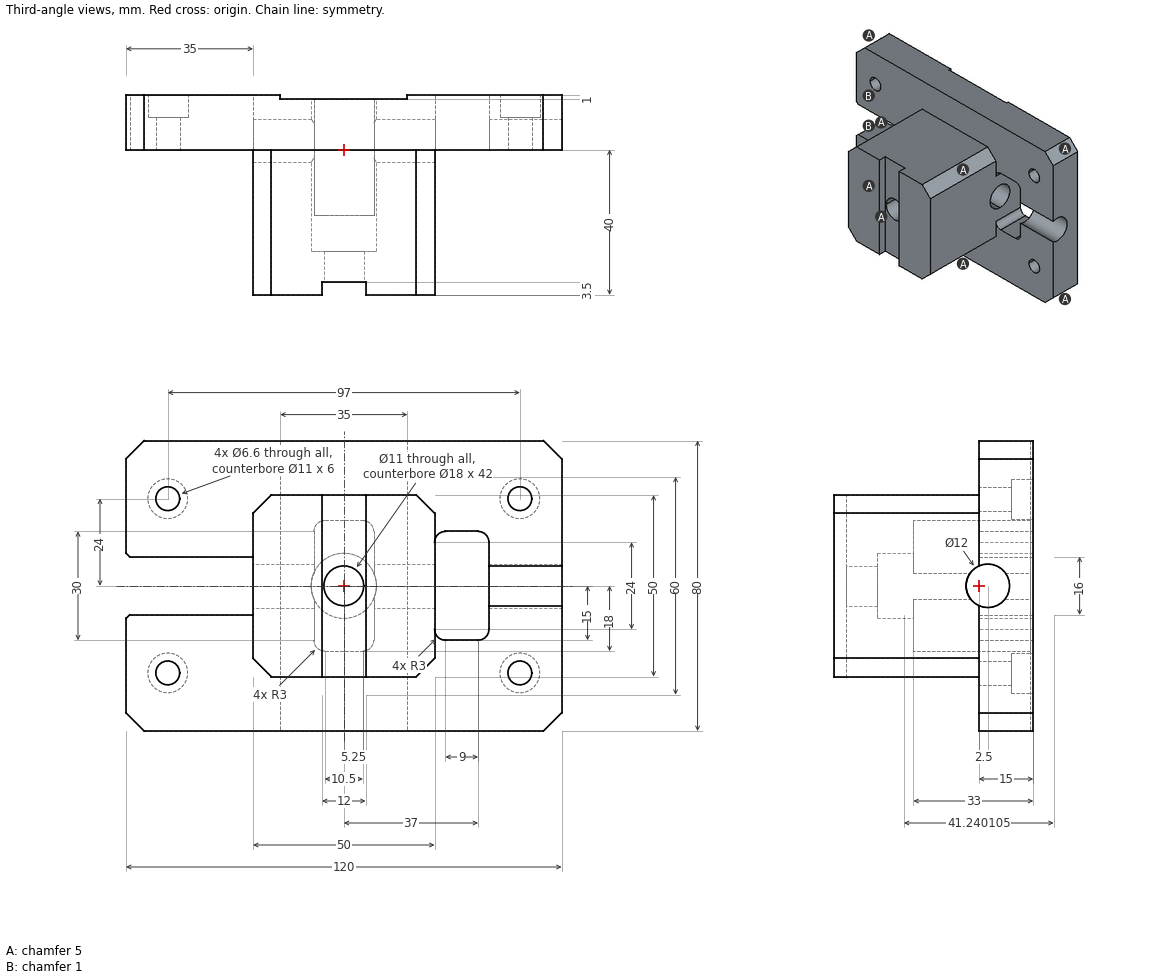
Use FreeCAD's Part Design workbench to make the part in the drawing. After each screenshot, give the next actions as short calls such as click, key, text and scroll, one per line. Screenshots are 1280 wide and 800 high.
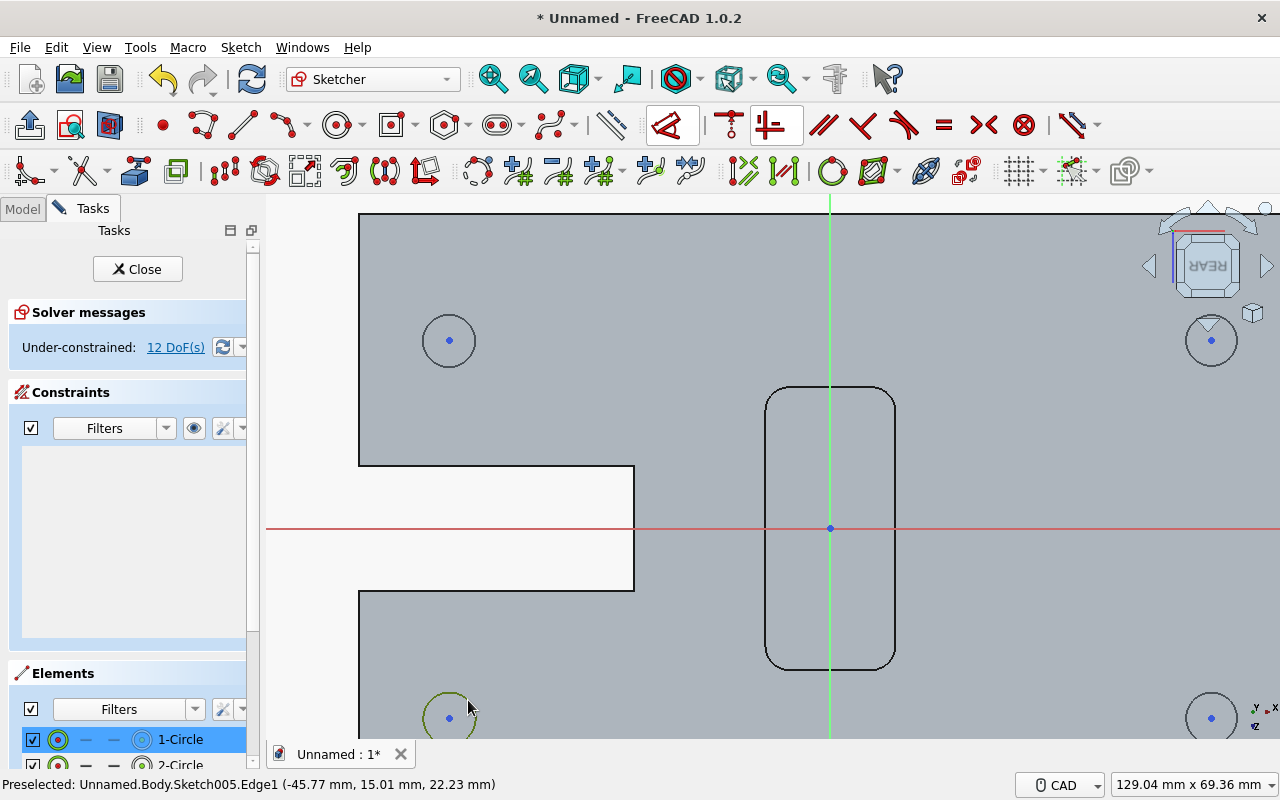
scroll(449, 340, down, 2)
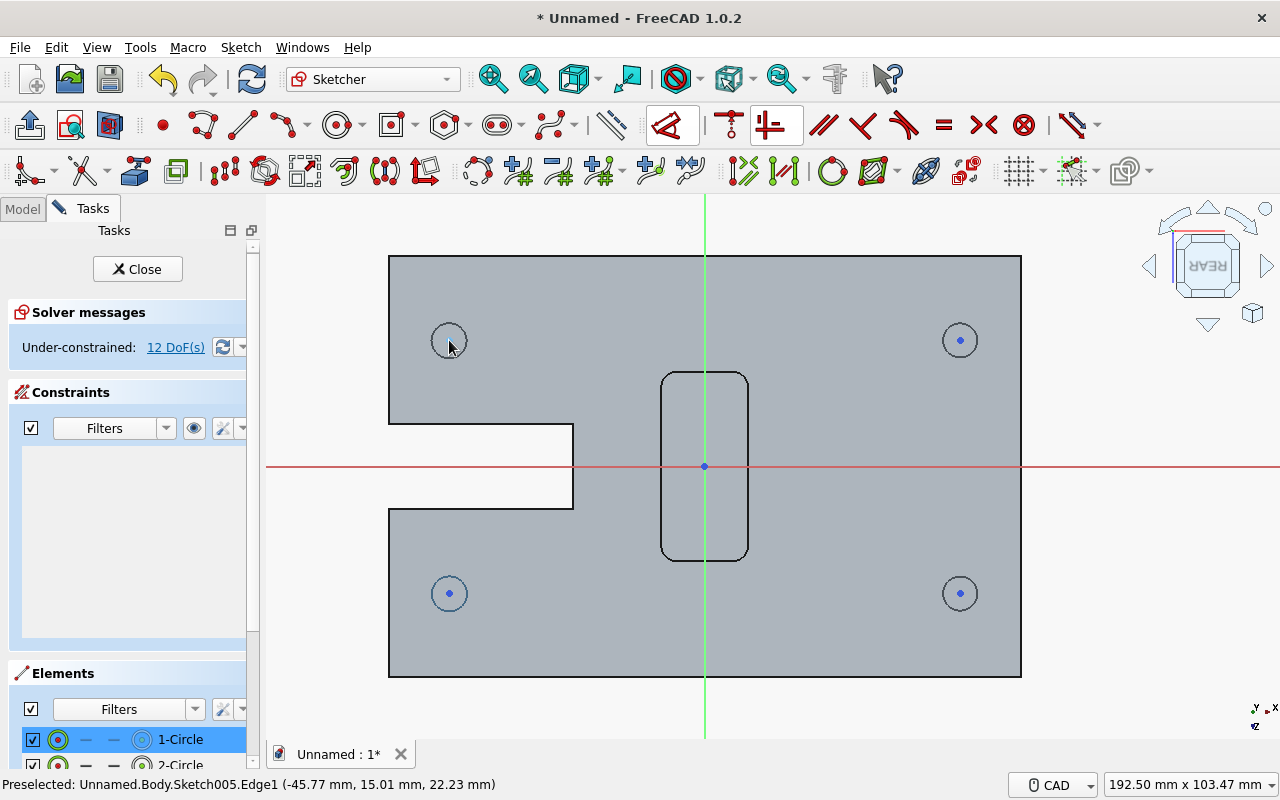
click(972, 581)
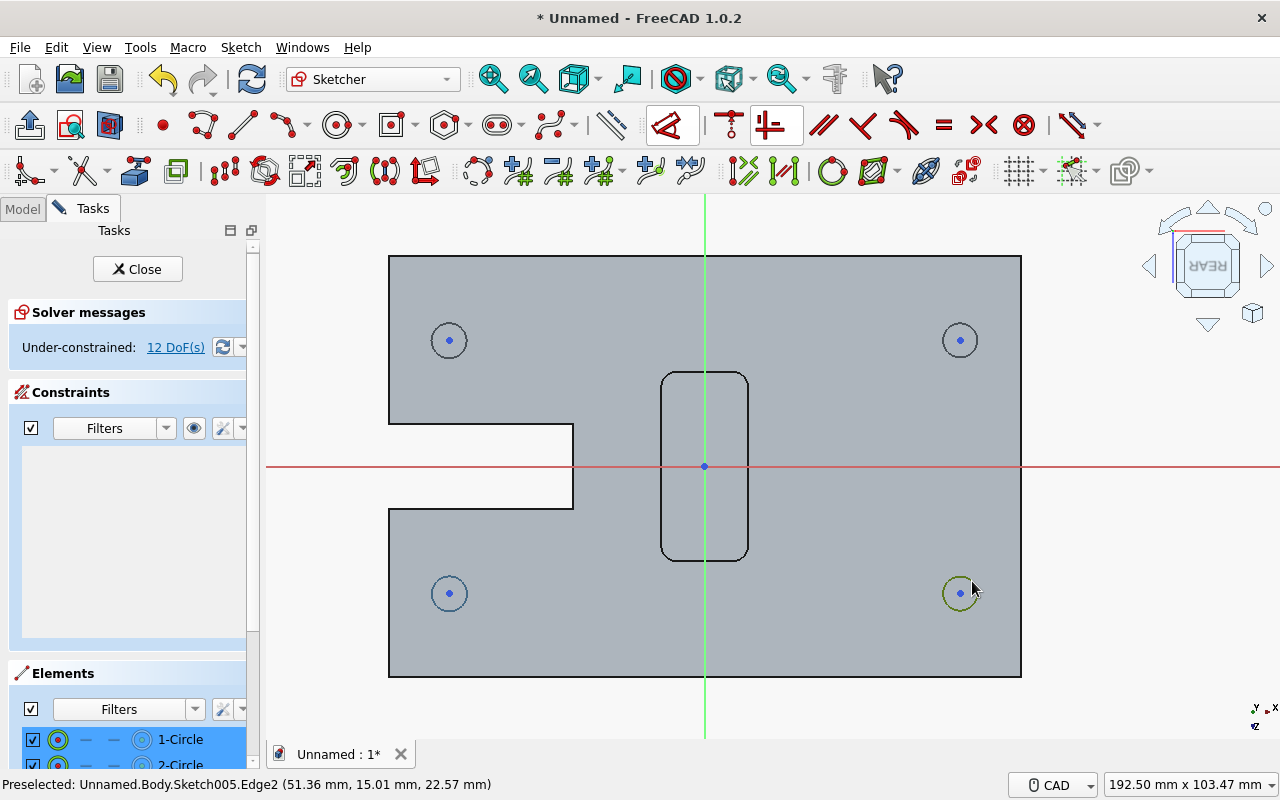
click(972, 328)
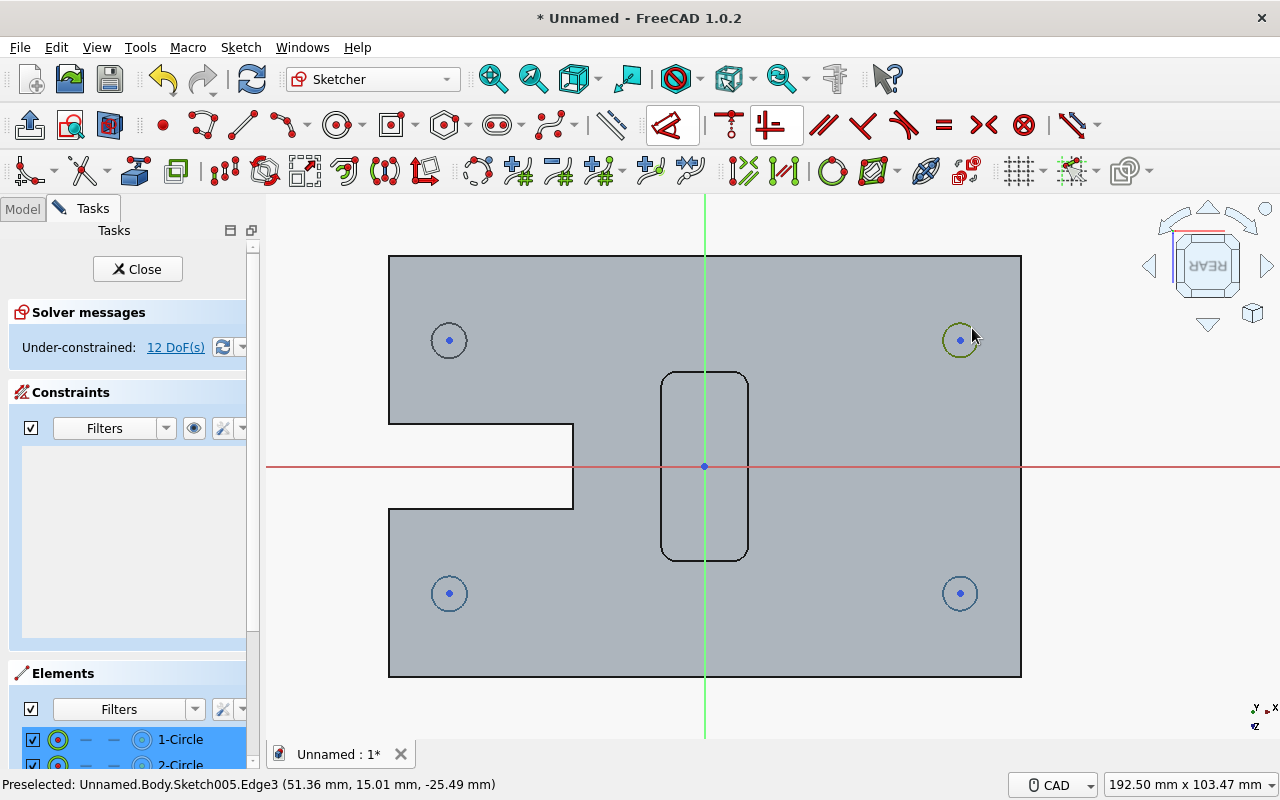
click(461, 328)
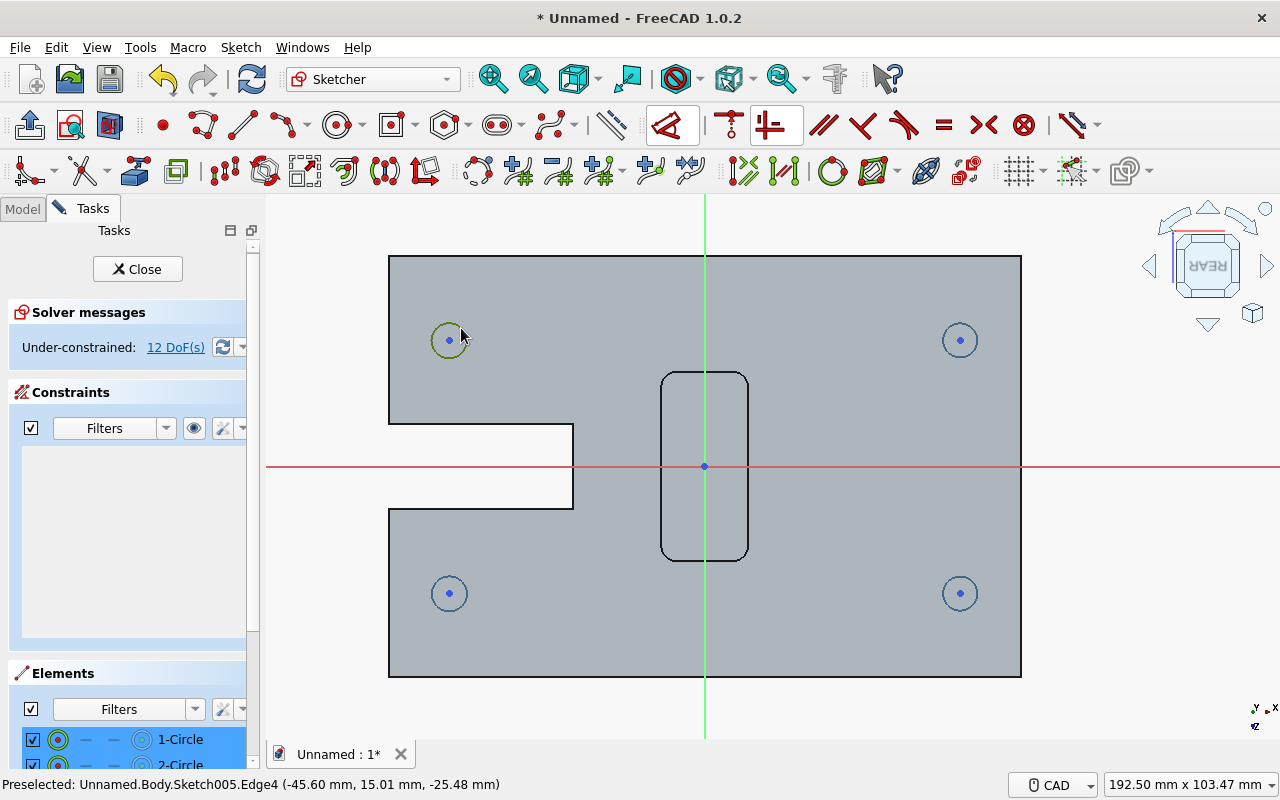
click(944, 126)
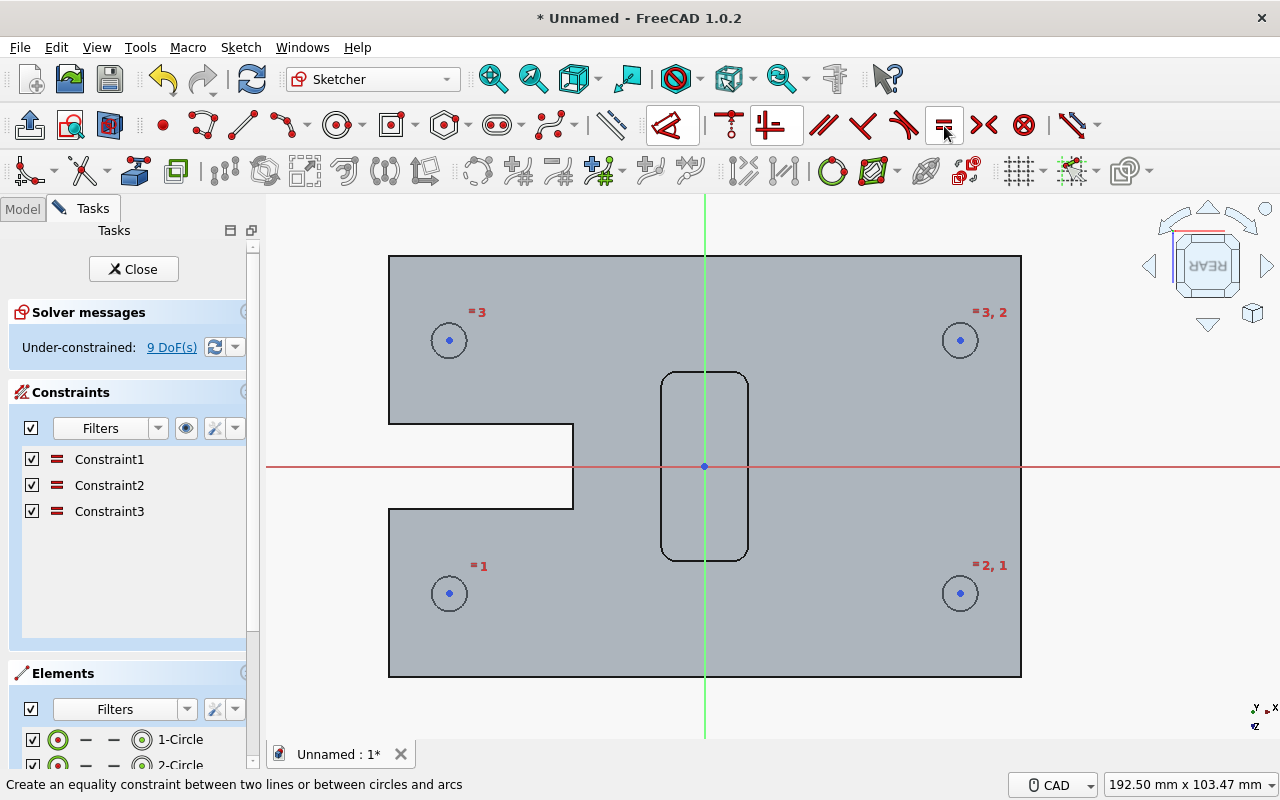
click(449, 594)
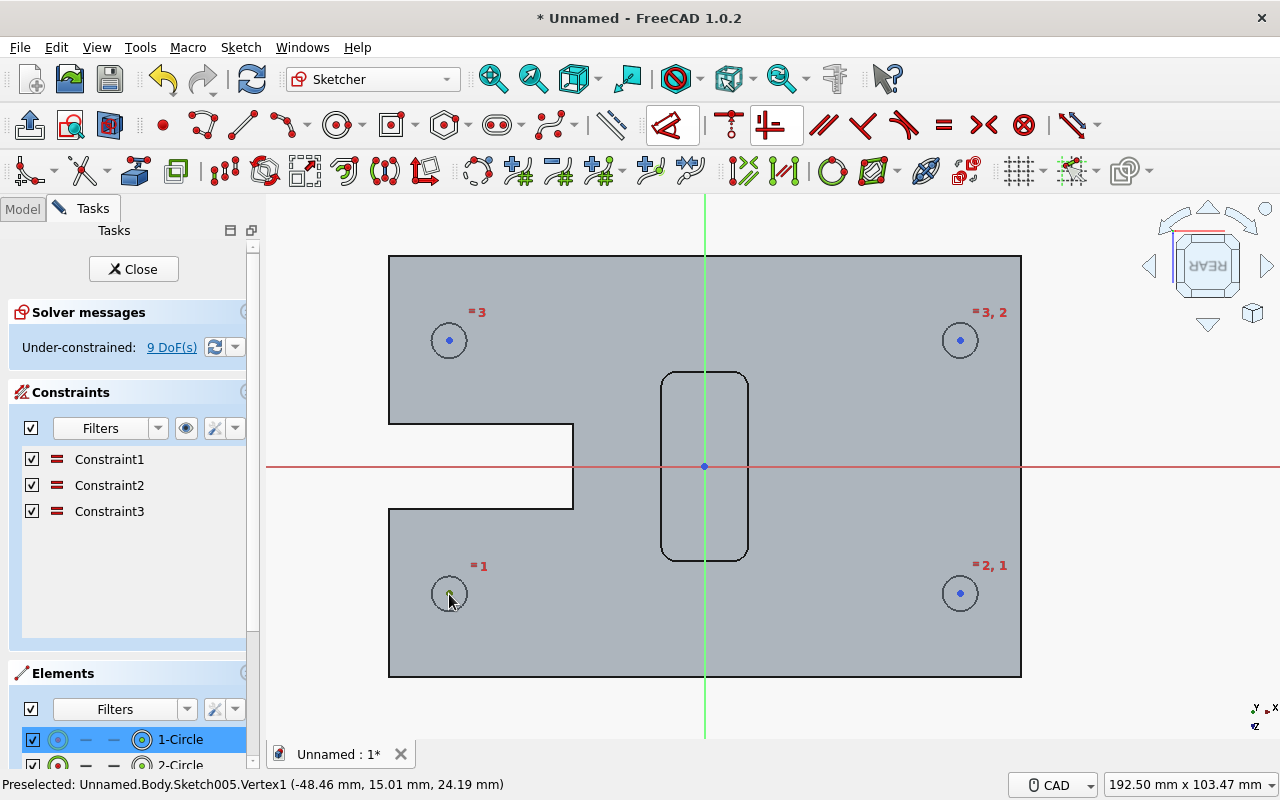
click(960, 594)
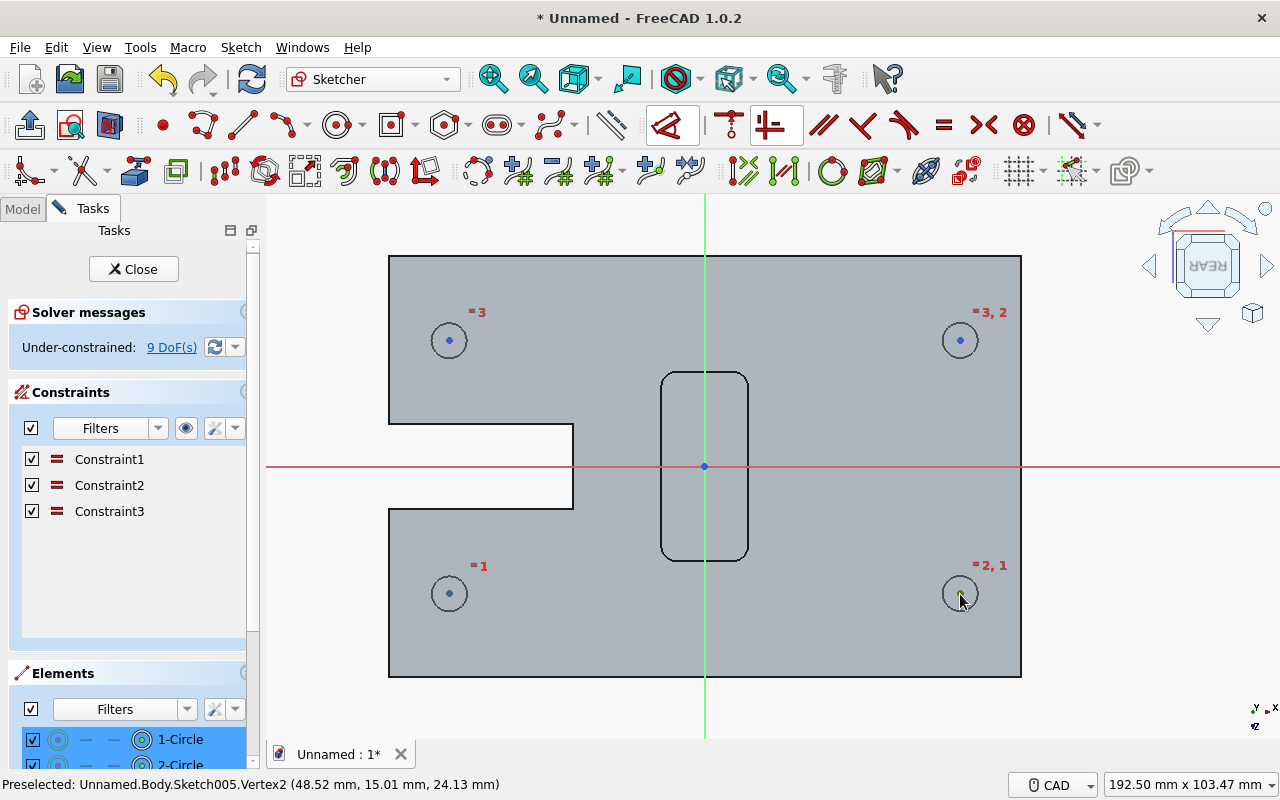
click(705, 676)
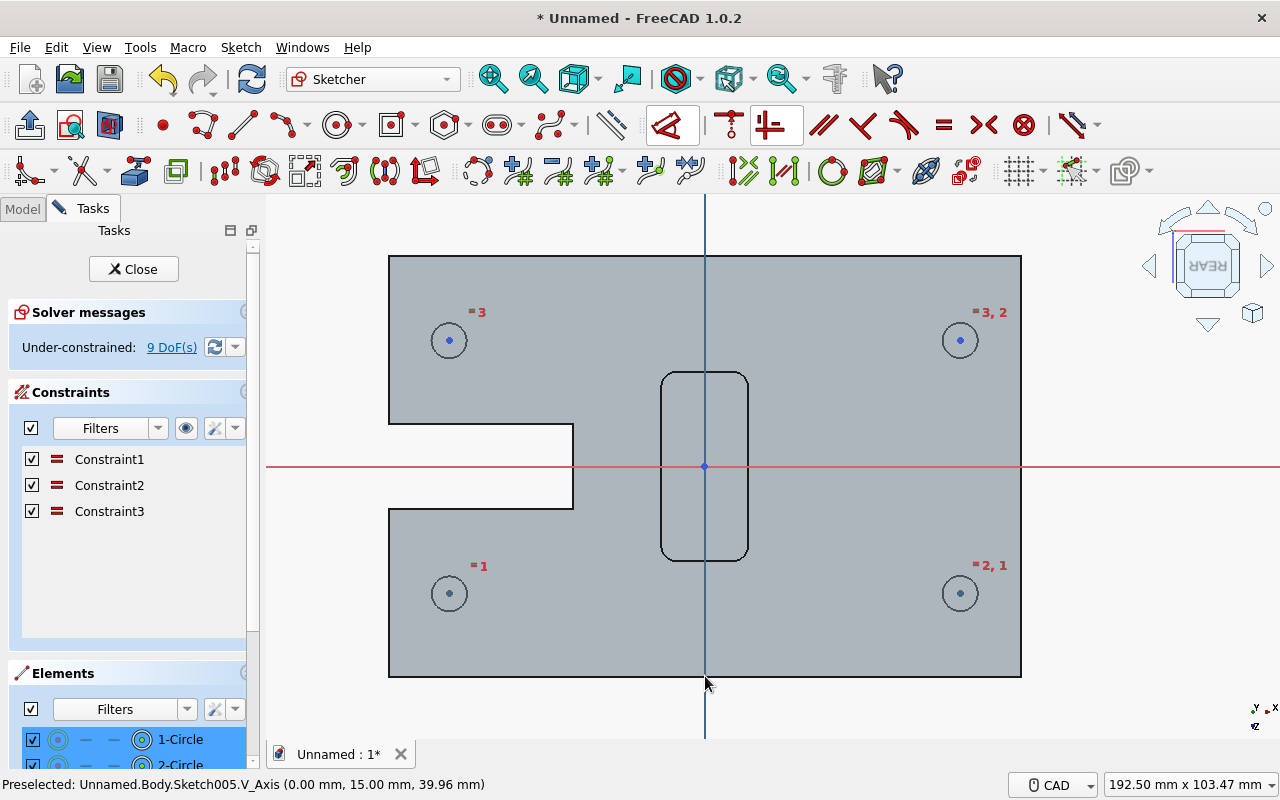
click(984, 126)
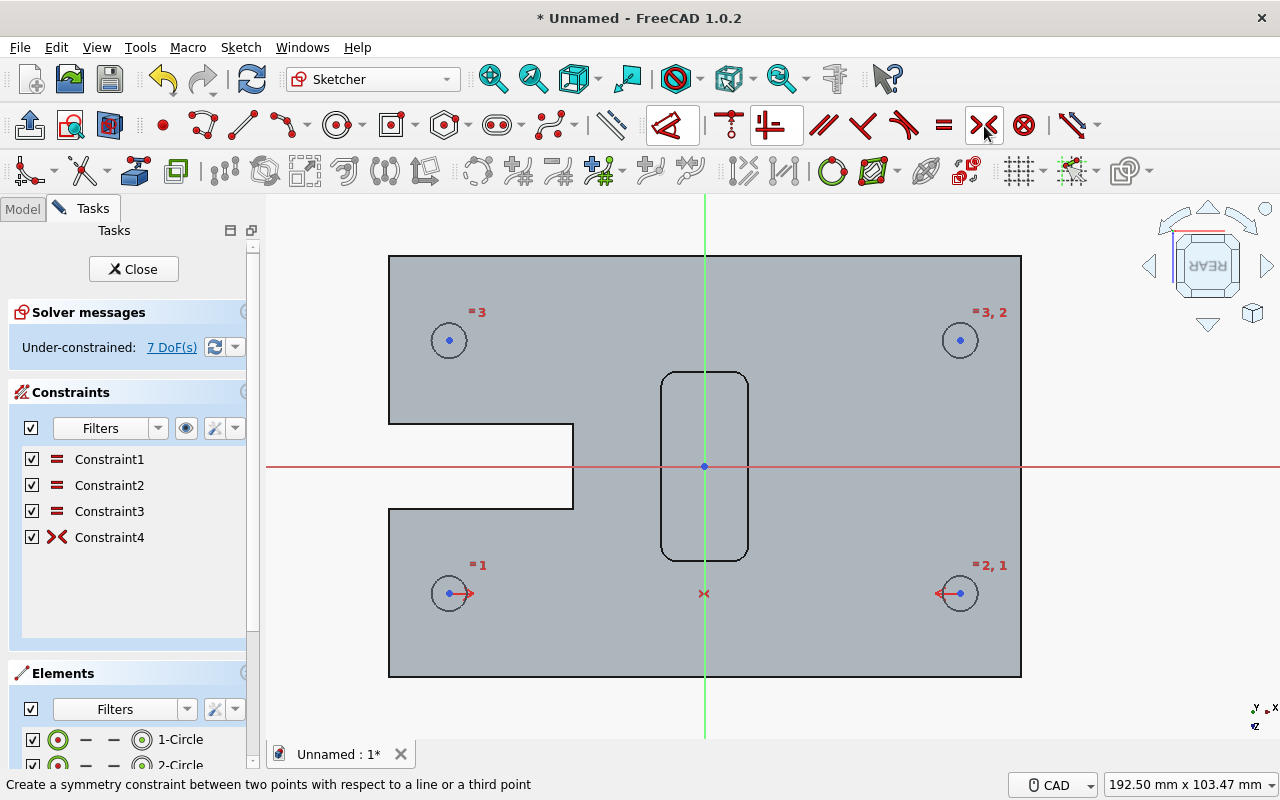
click(960, 594)